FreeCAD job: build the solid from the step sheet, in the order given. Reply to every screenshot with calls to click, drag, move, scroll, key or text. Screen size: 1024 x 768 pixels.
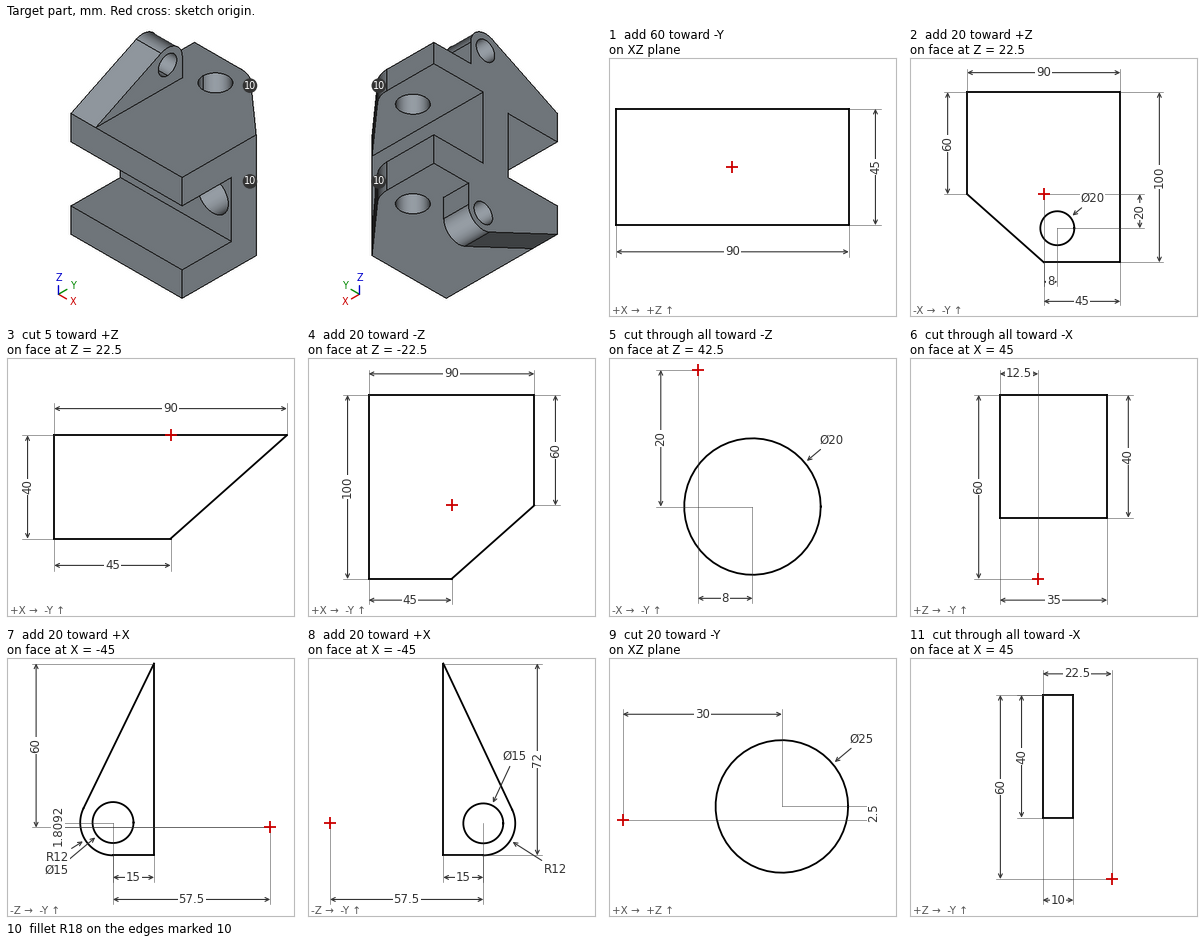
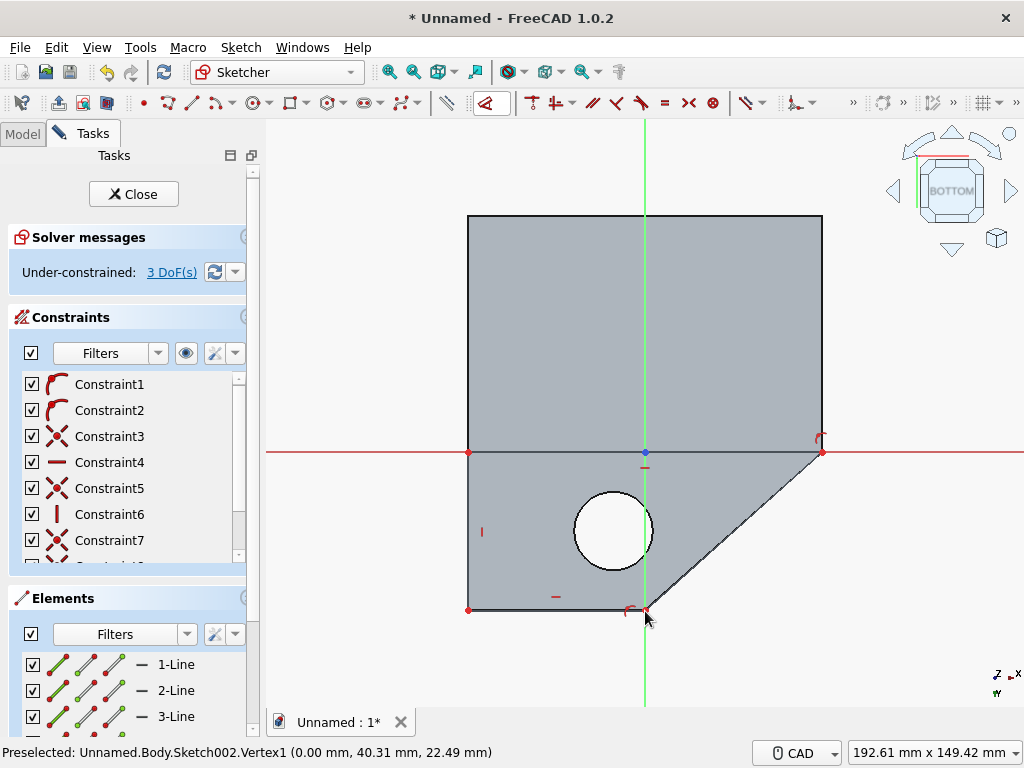
click(716, 452)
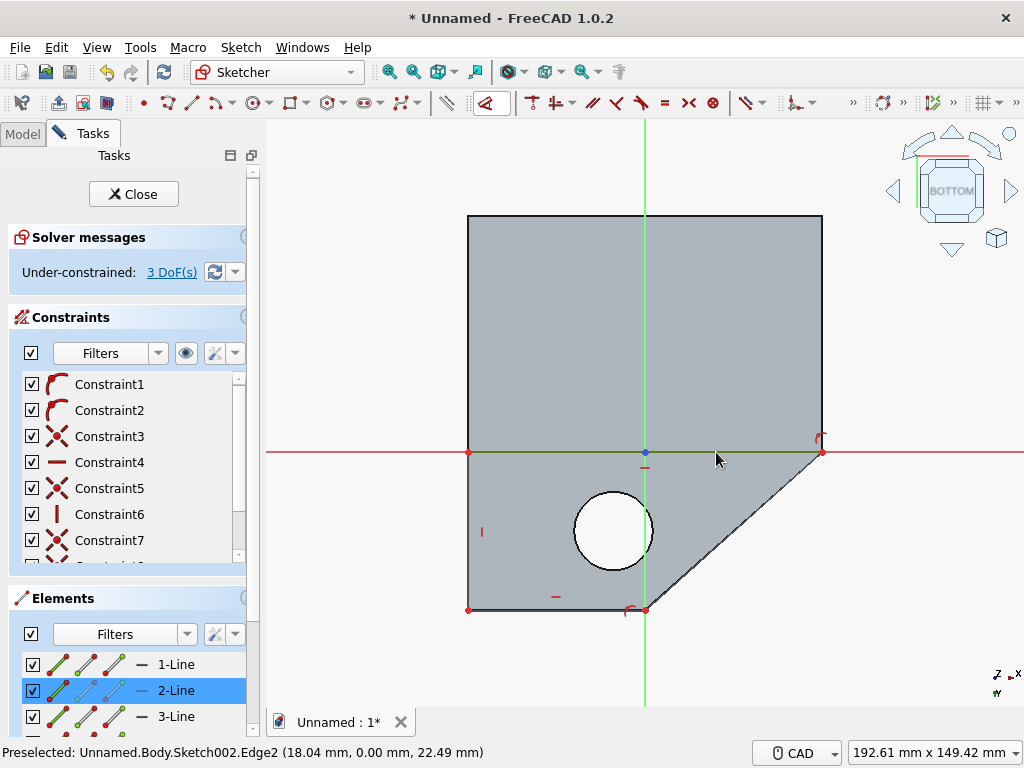
key(l)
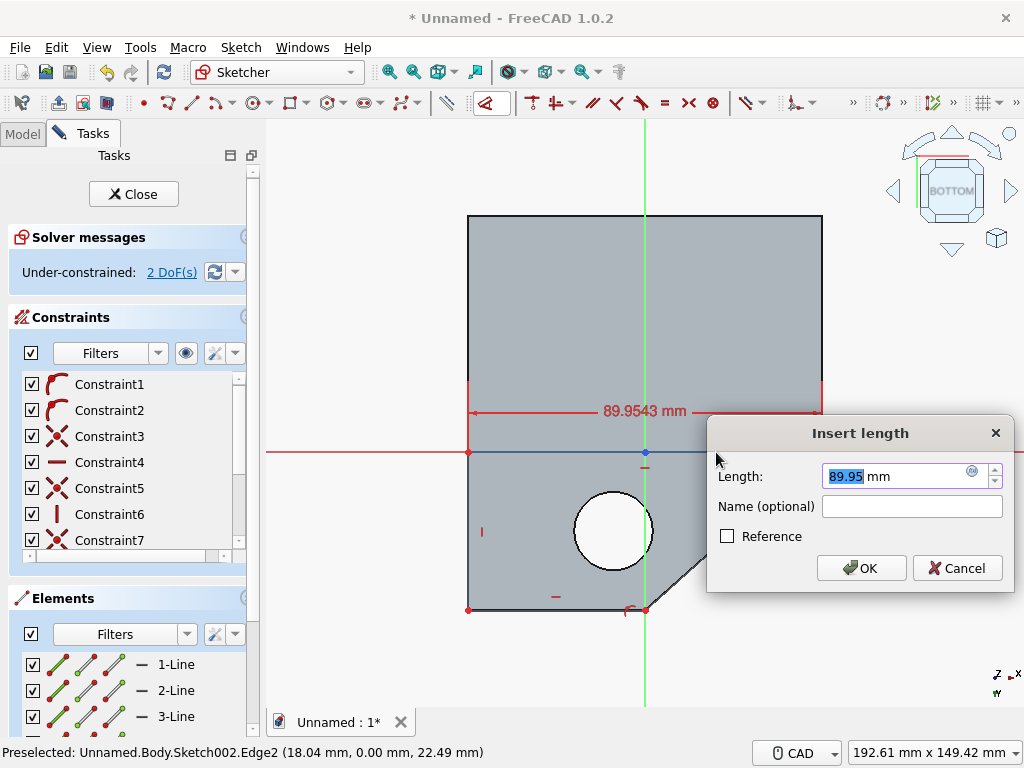
text(90)
key(Return)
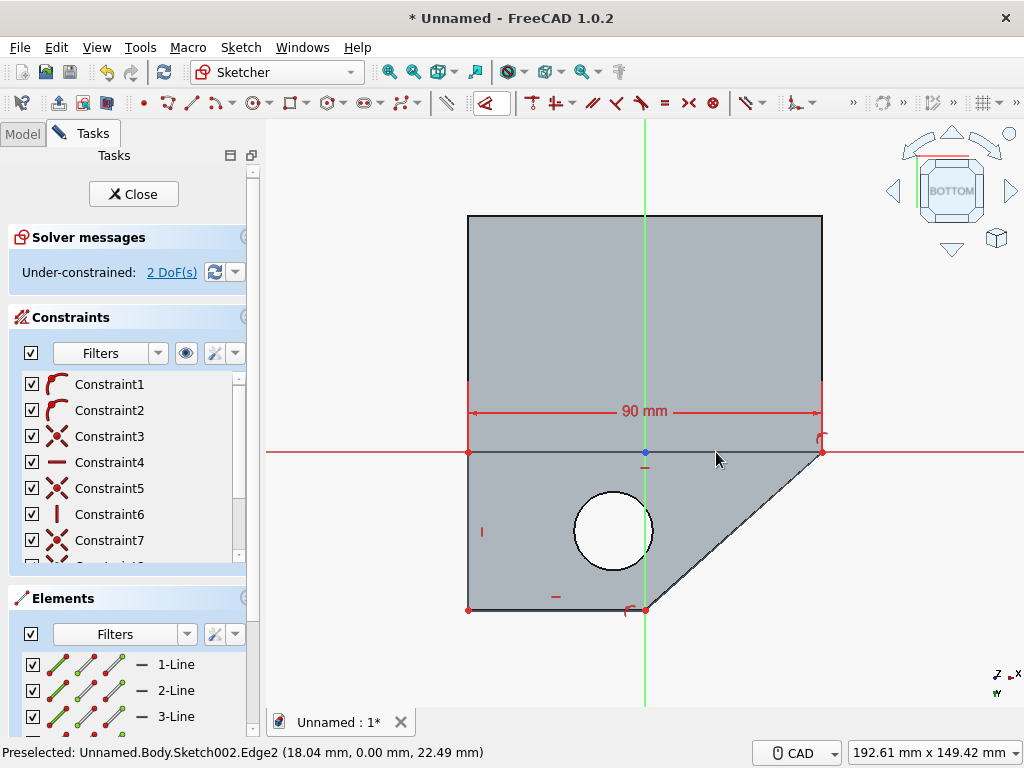
click(468, 500)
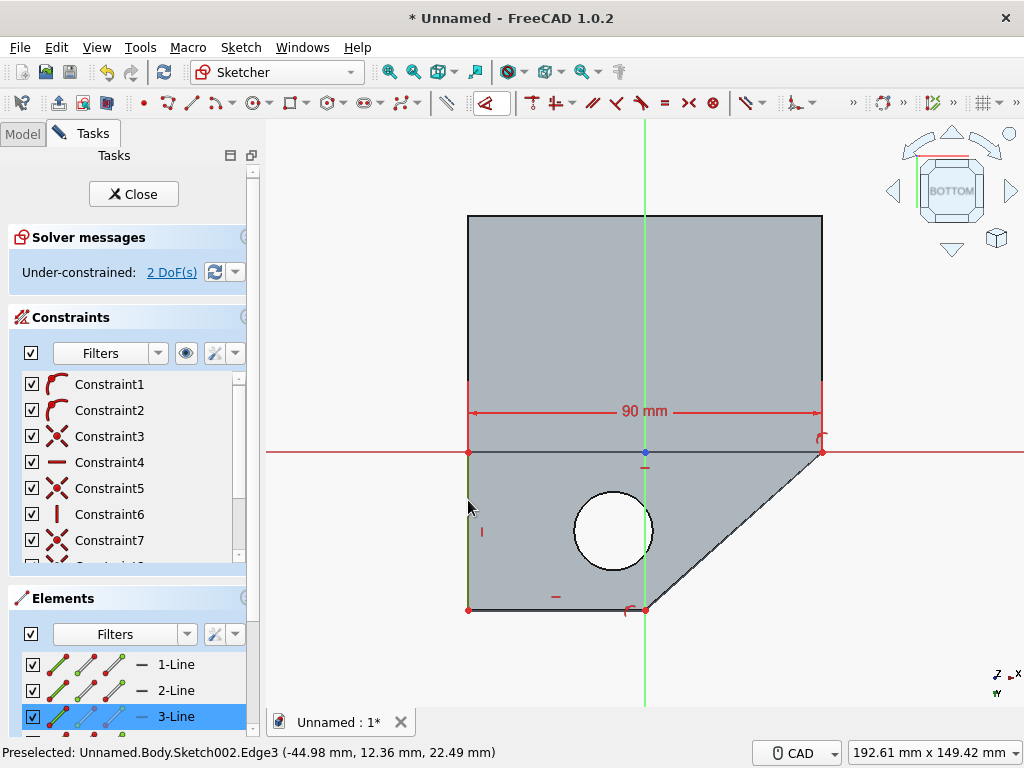
key(i)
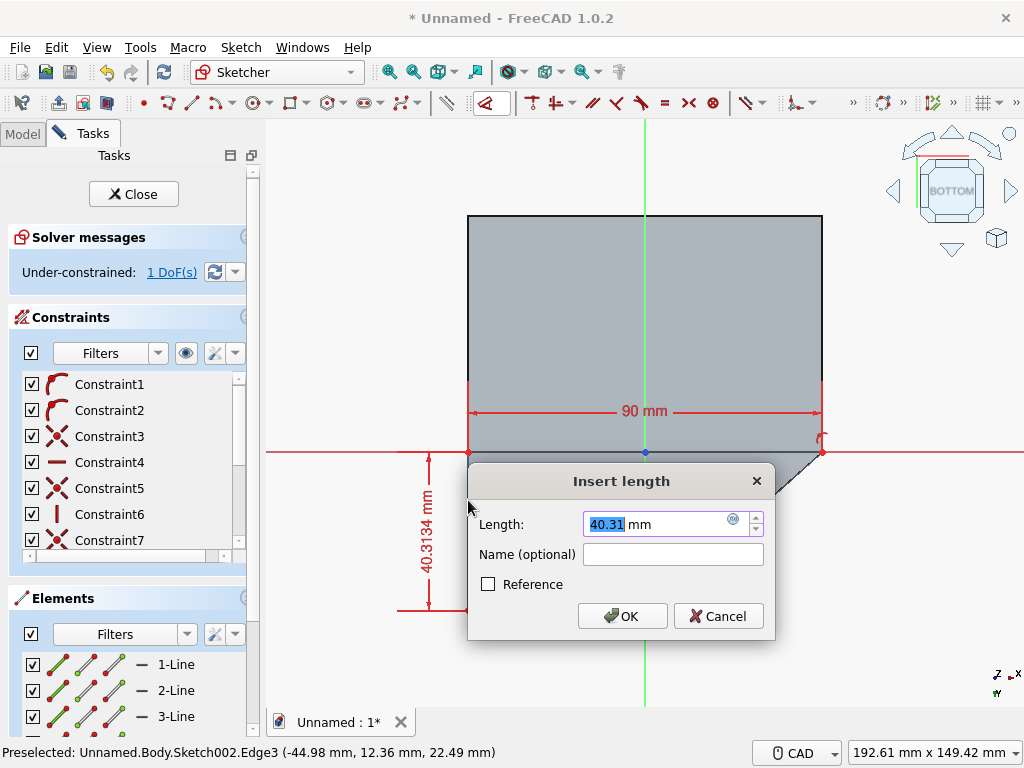
text(40)
key(Return)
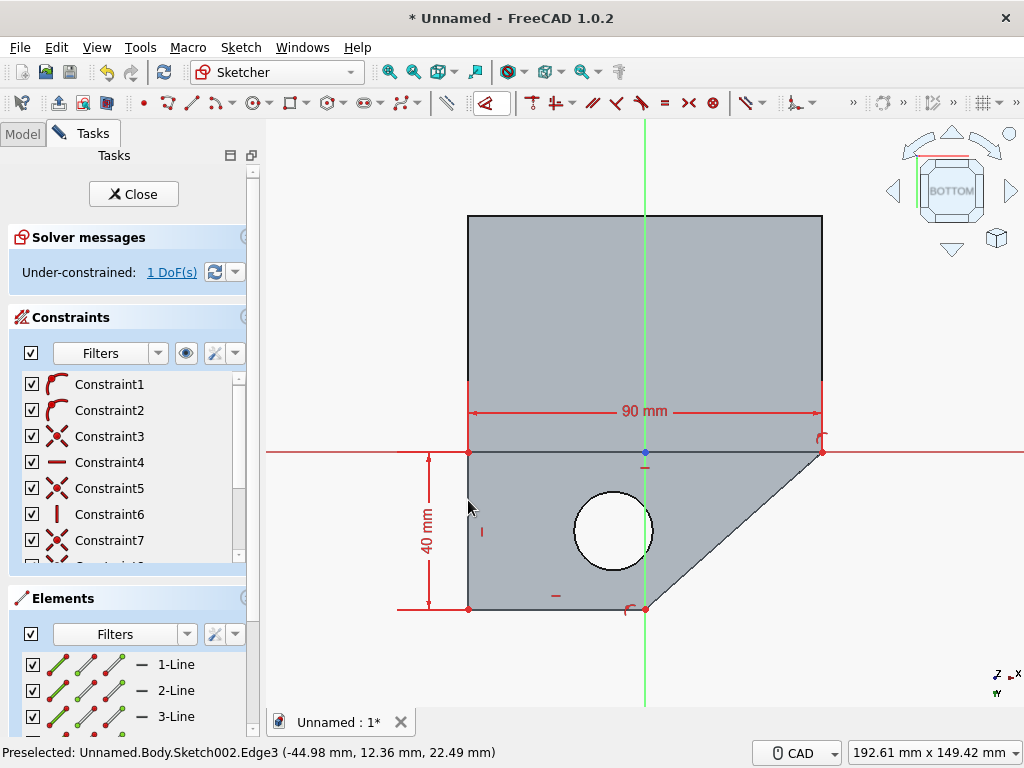
click(521, 610)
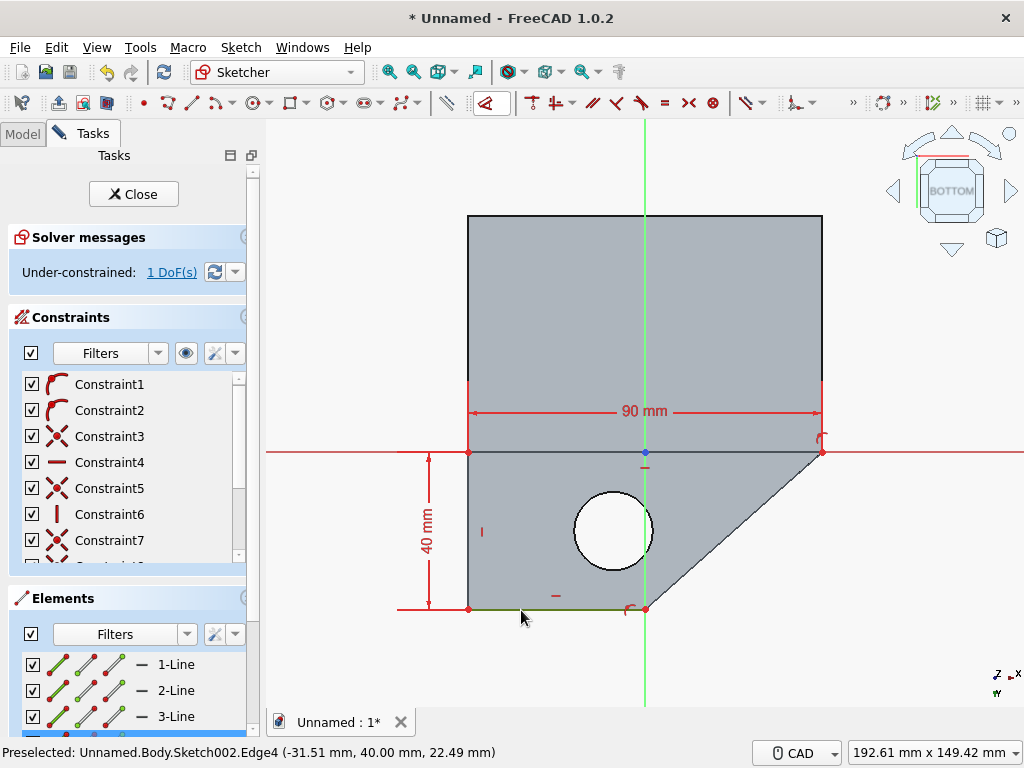
key(l)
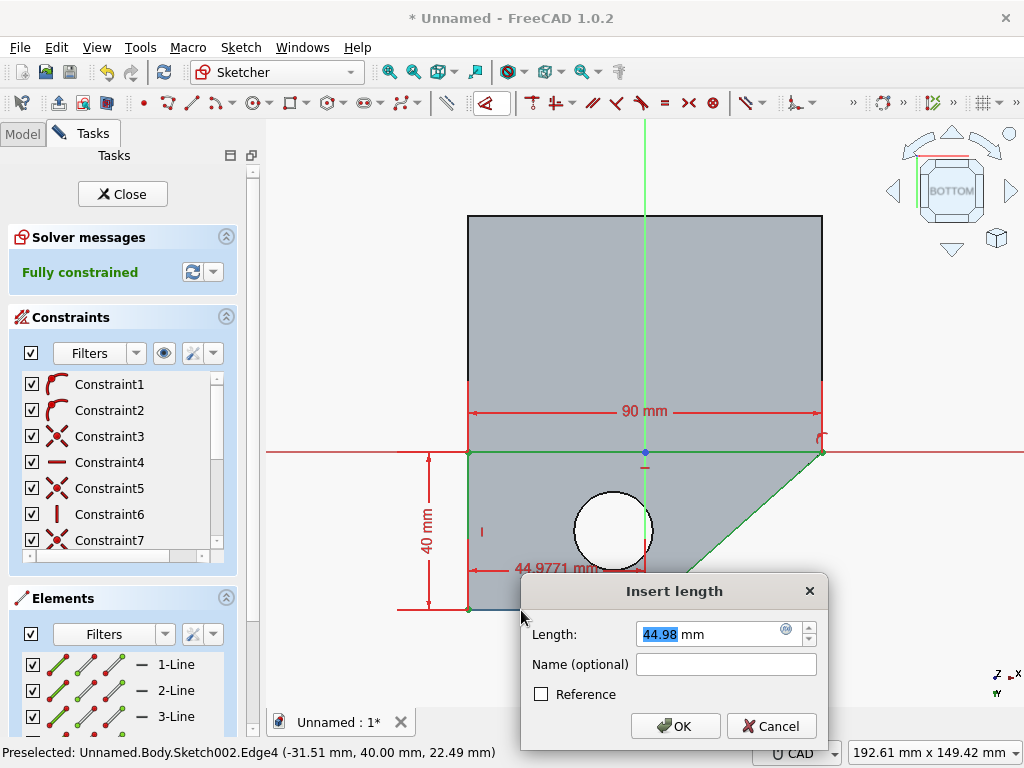
text(45)
key(Return)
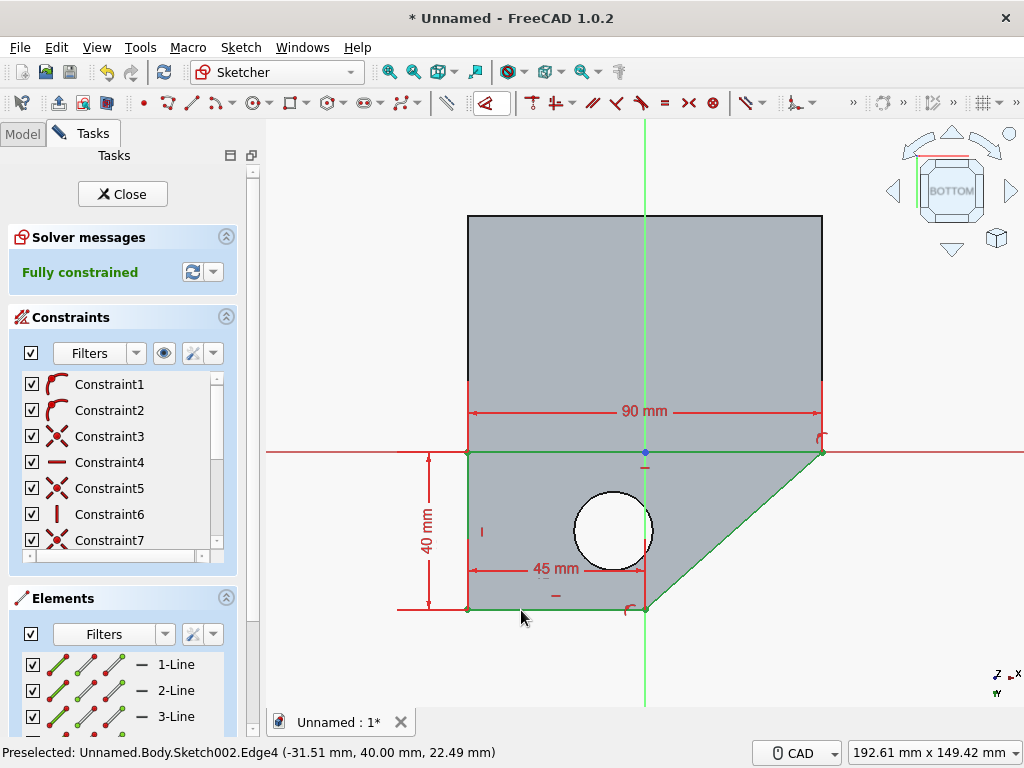
click(123, 194)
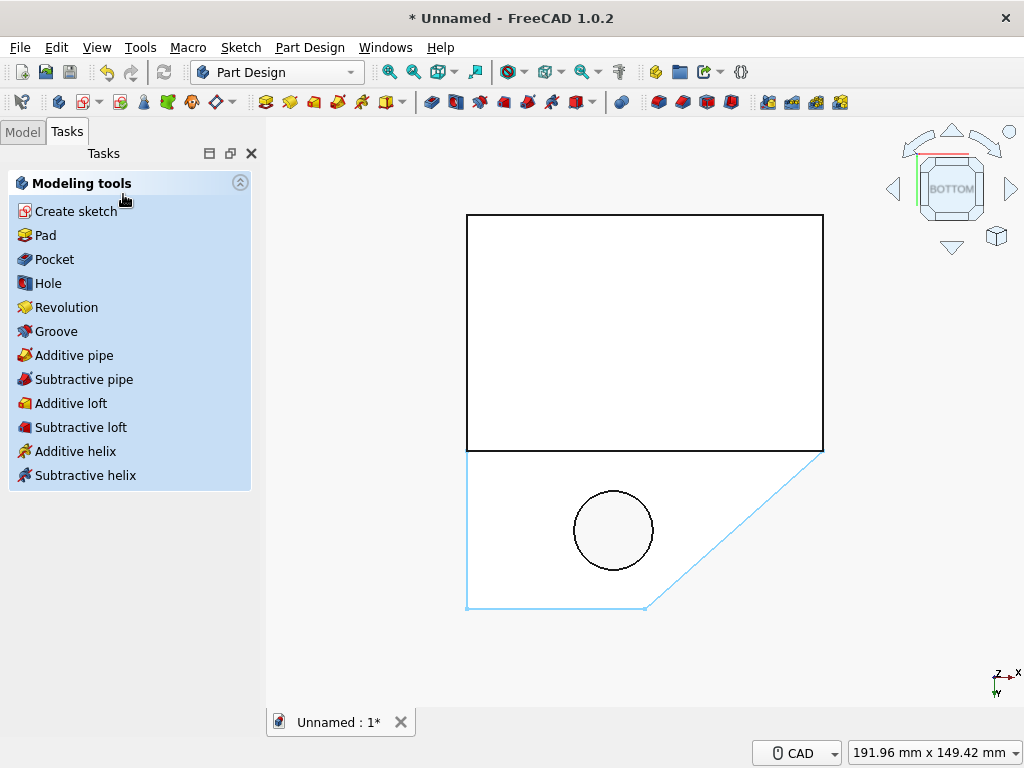
click(432, 102)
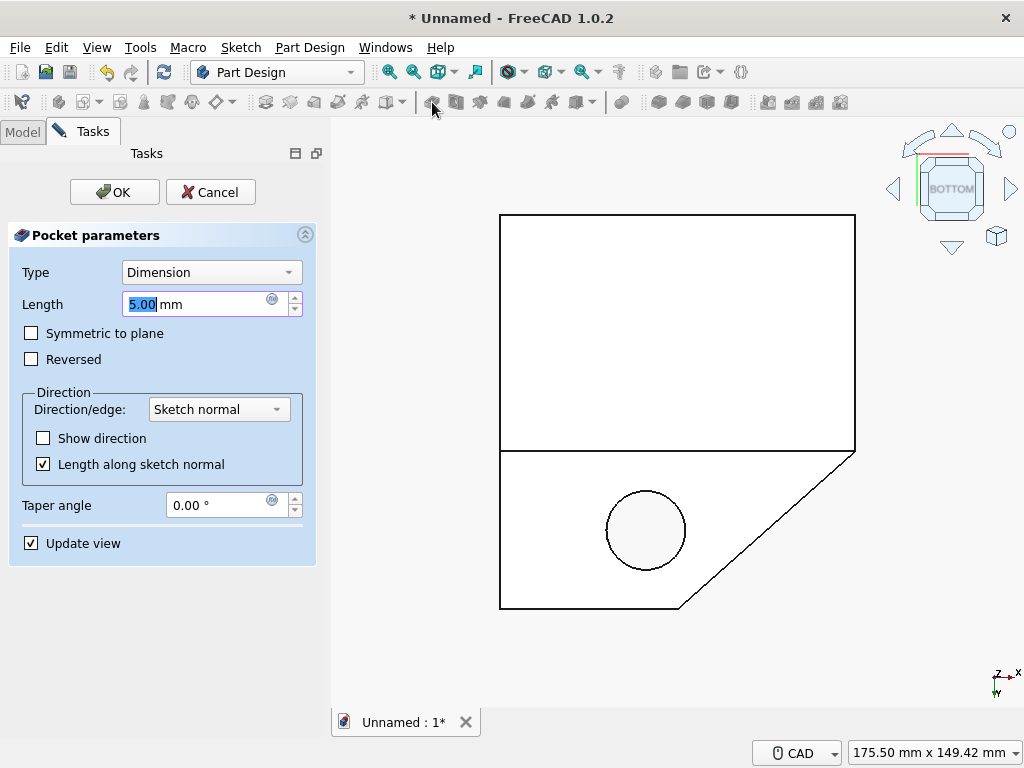
text(5)
key(Tab)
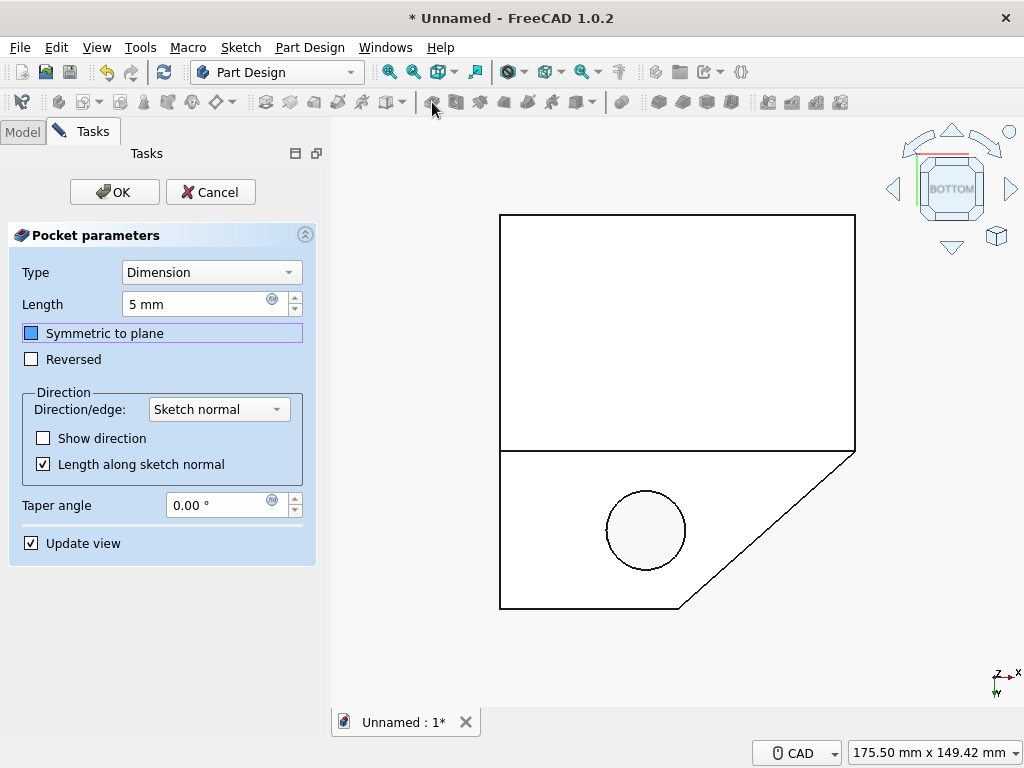
click(115, 192)